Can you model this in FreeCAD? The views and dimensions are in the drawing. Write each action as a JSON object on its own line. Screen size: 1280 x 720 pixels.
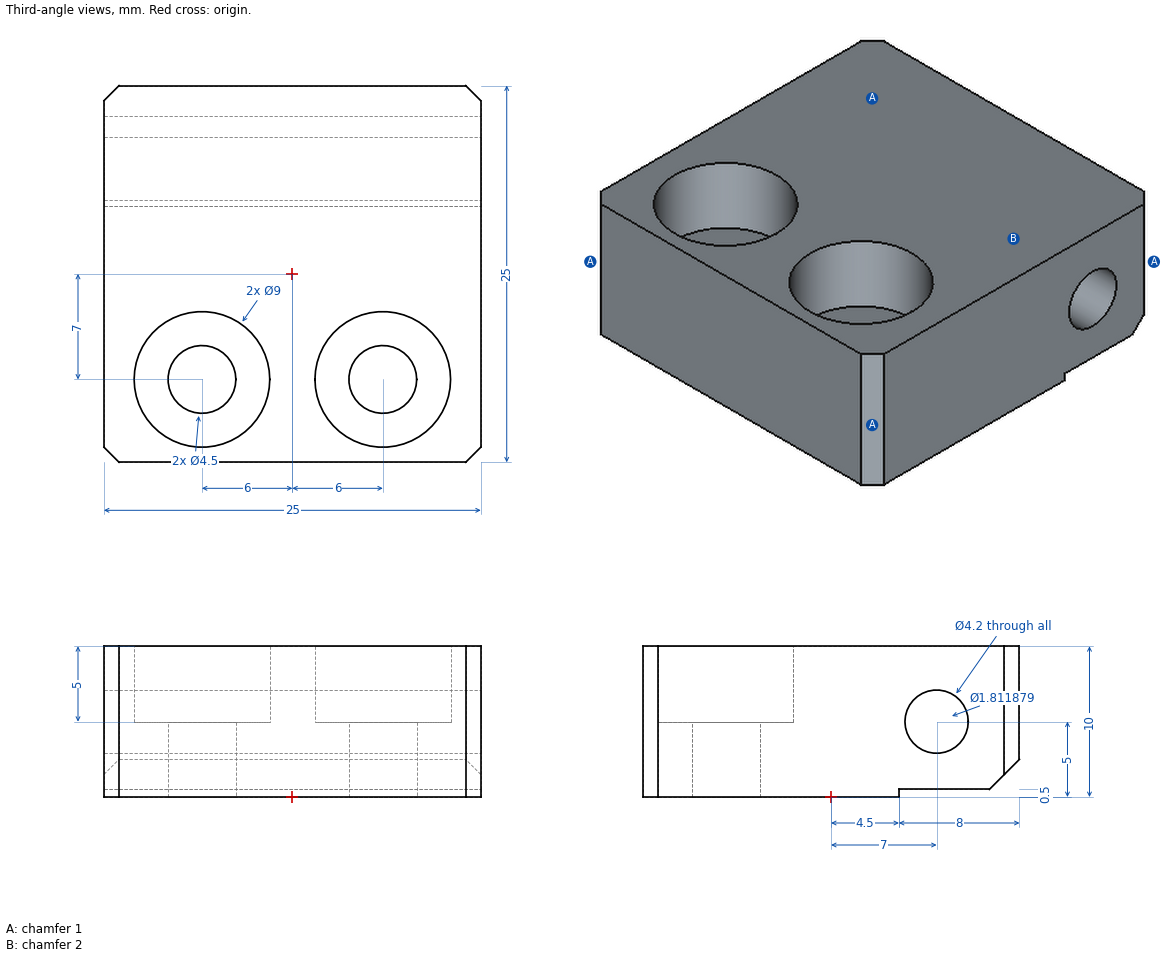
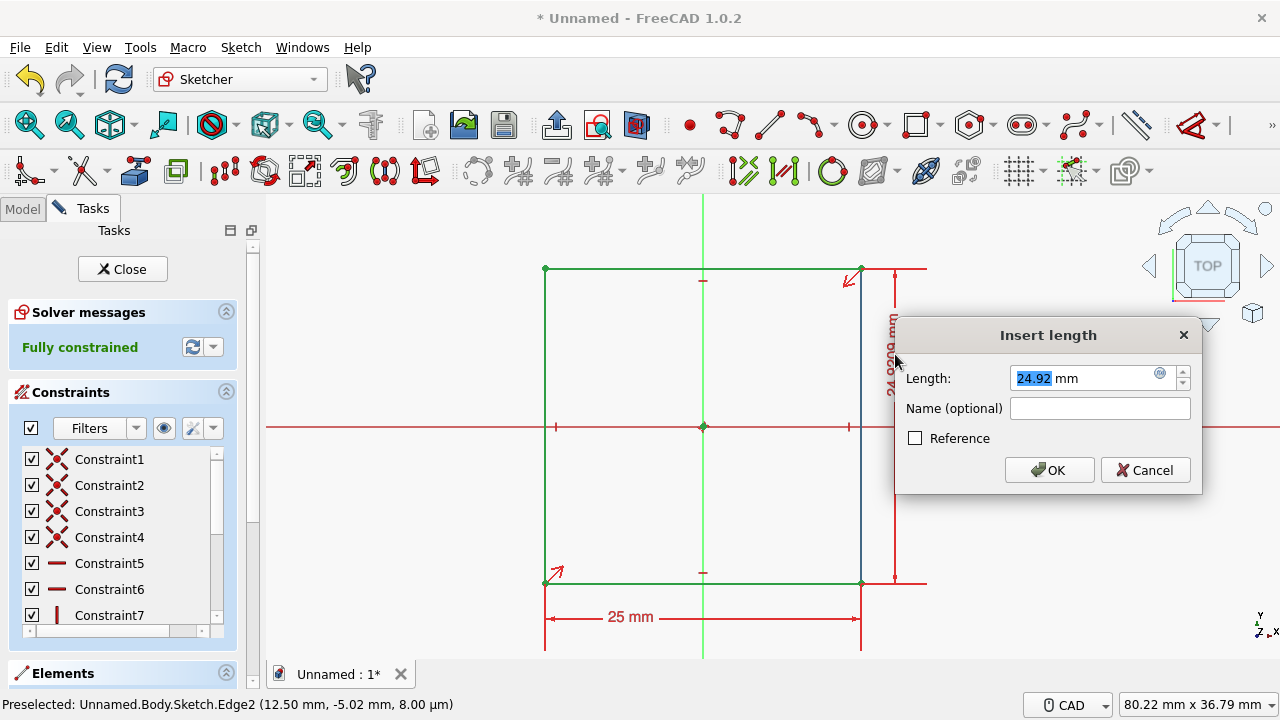
{"action": "type", "text": "25"}
{"action": "key", "text": "Return"}
{"action": "key", "text": "Escape"}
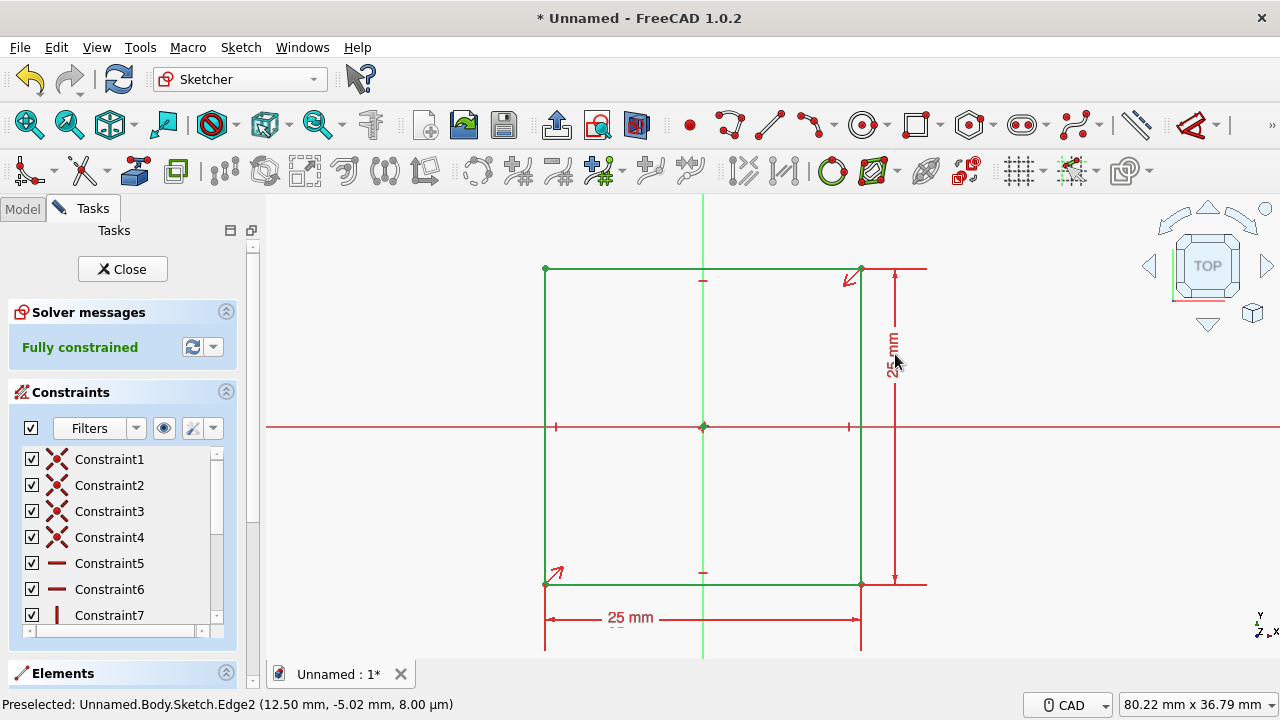
{"action": "left_click", "coordinate": [123, 269]}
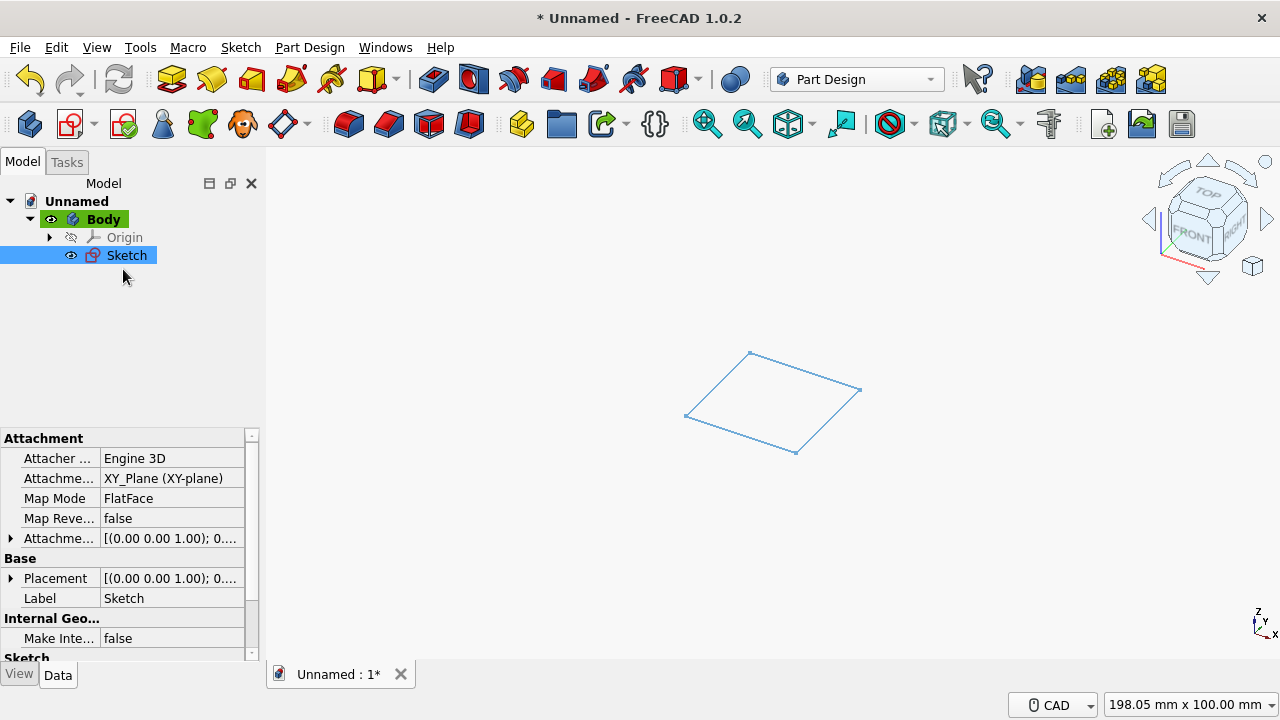
{"action": "left_click", "coordinate": [172, 80]}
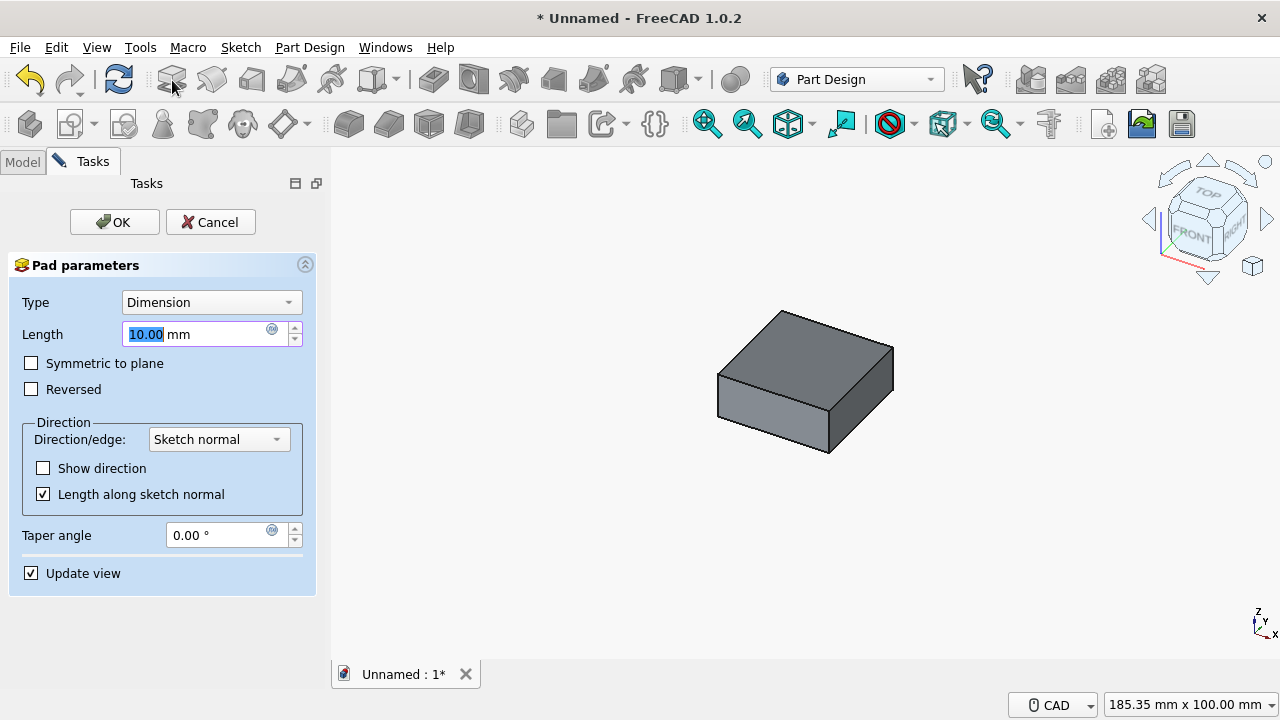
{"action": "type", "text": "10"}
{"action": "key", "text": "Tab"}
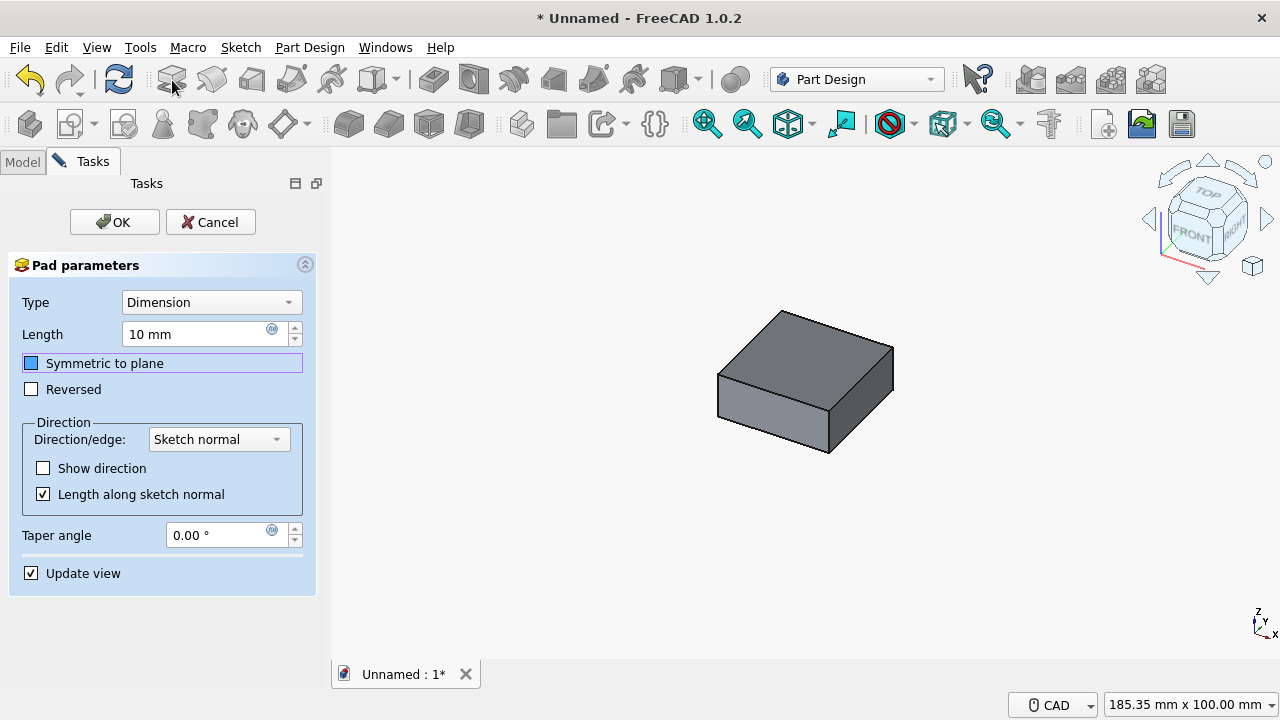
{"action": "left_click", "coordinate": [115, 222]}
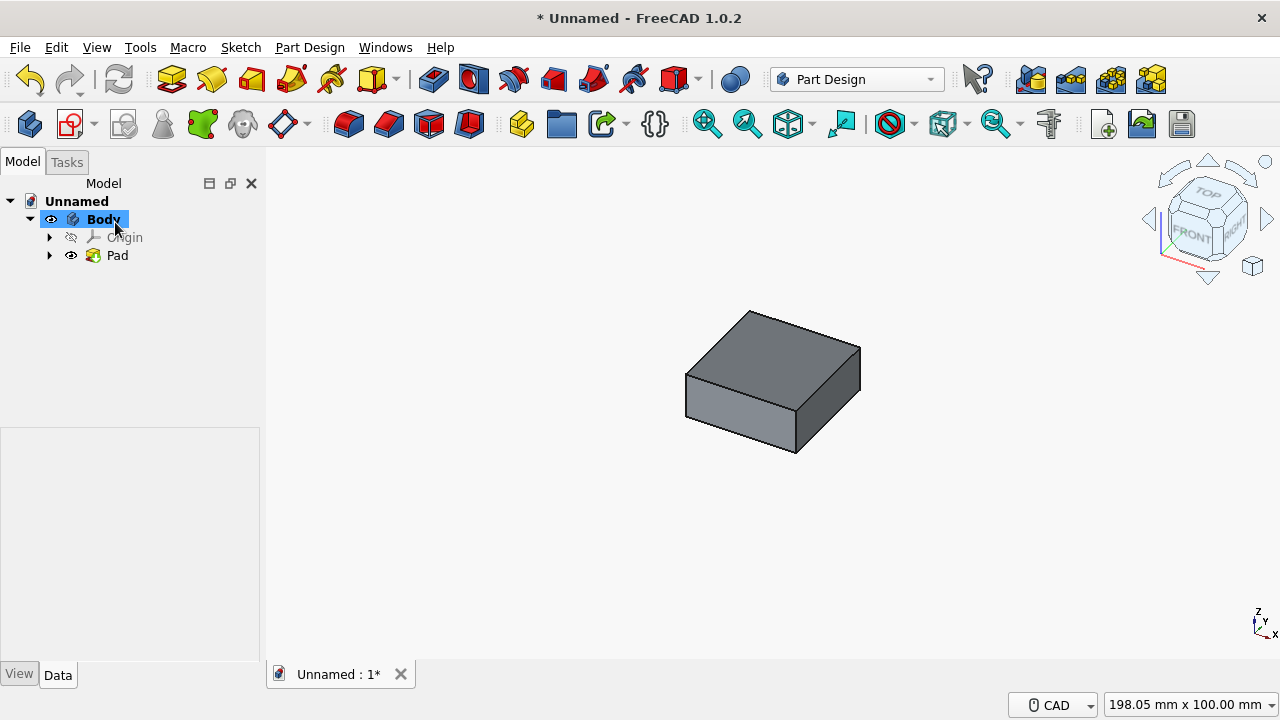
{"action": "key", "text": "v f"}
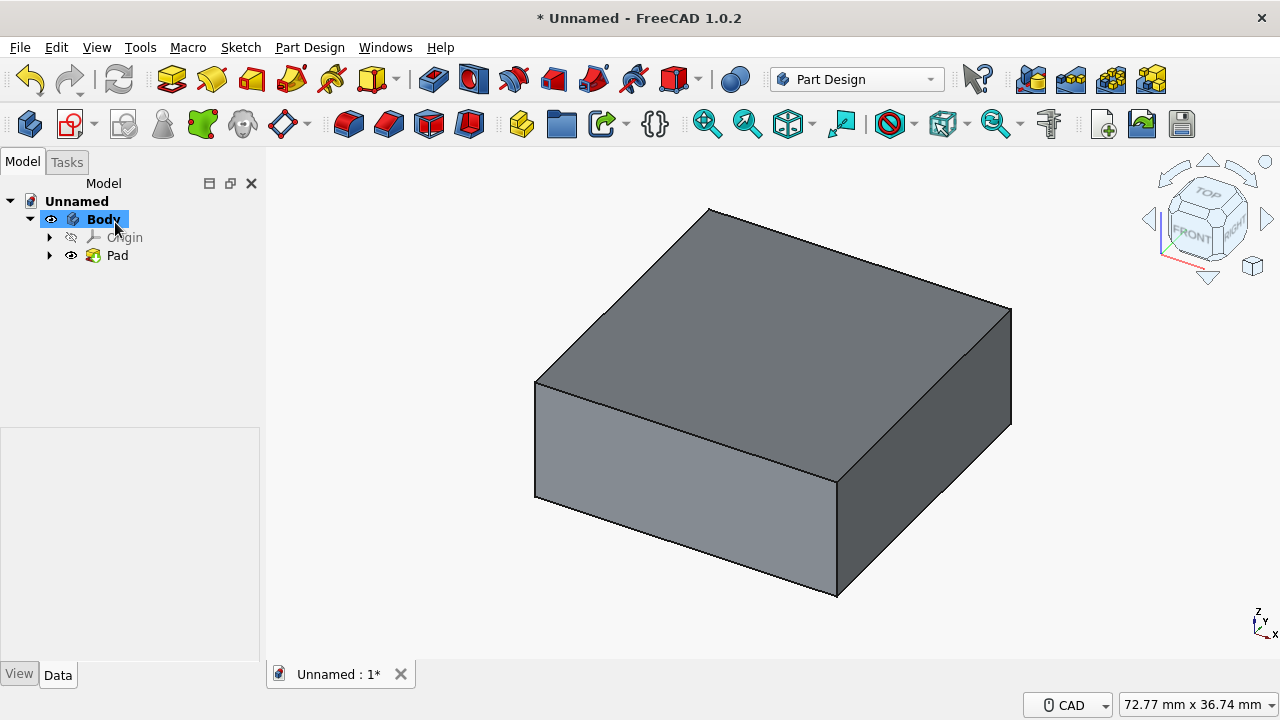
{"action": "left_click", "coordinate": [773, 345]}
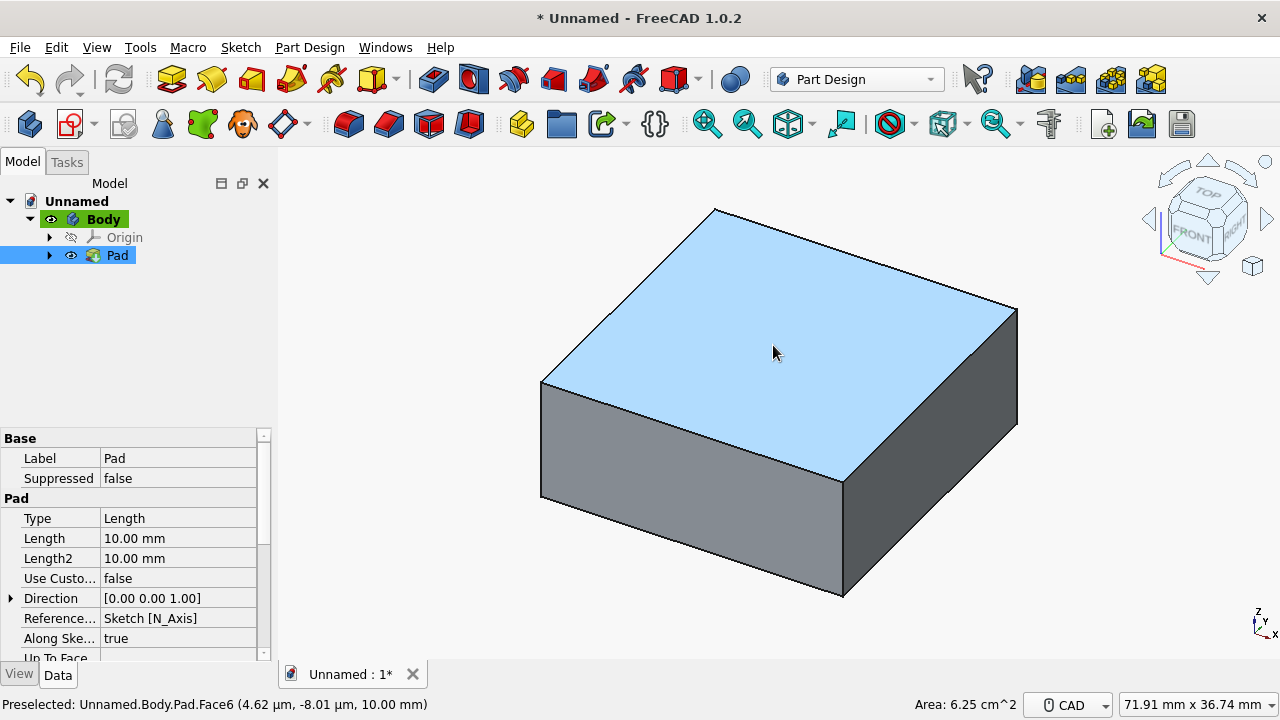
{"action": "left_click", "coordinate": [70, 124]}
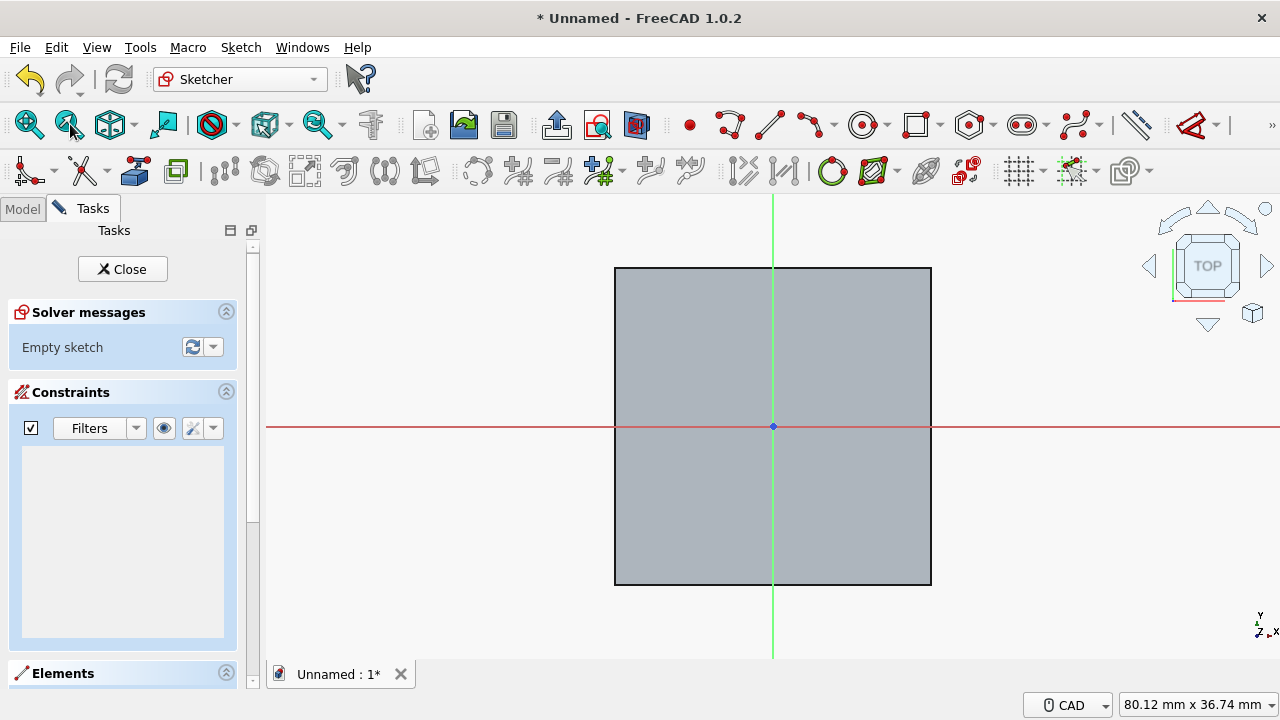
{"action": "scroll", "coordinate": [856, 588], "scroll_direction": "up", "scroll_amount": 3}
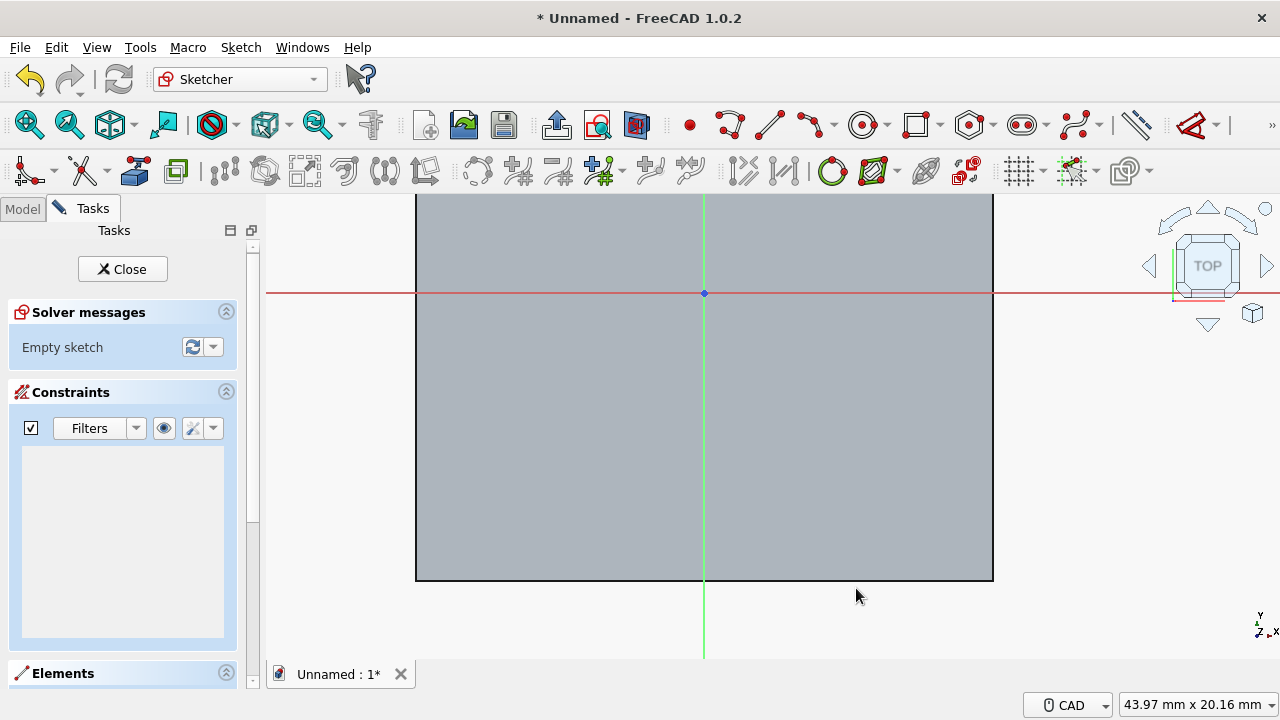
{"action": "key", "text": "g c"}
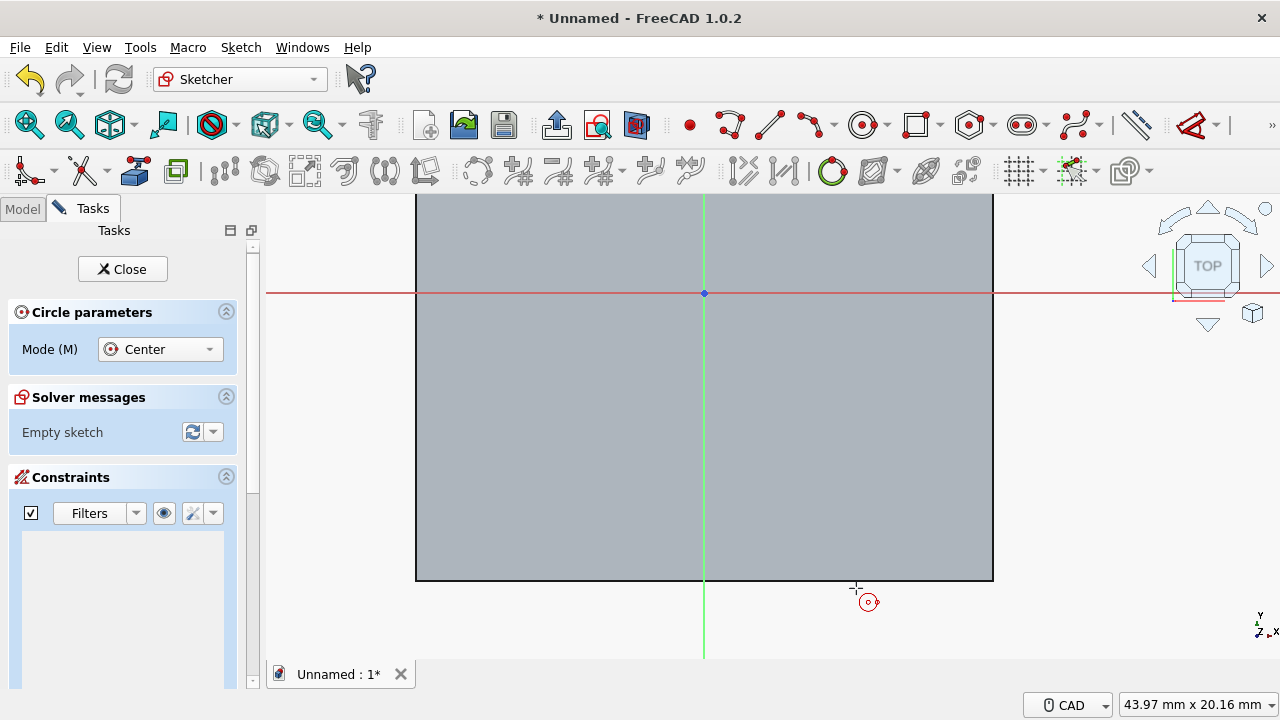
{"action": "left_click", "coordinate": [566, 454]}
{"action": "left_click", "coordinate": [639, 381]}